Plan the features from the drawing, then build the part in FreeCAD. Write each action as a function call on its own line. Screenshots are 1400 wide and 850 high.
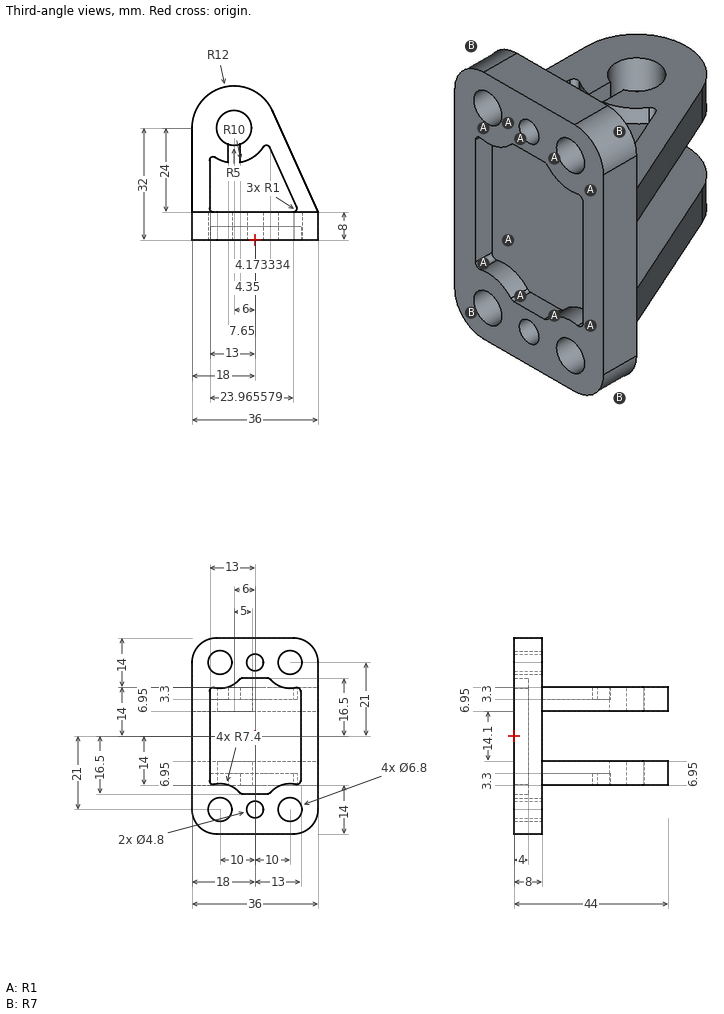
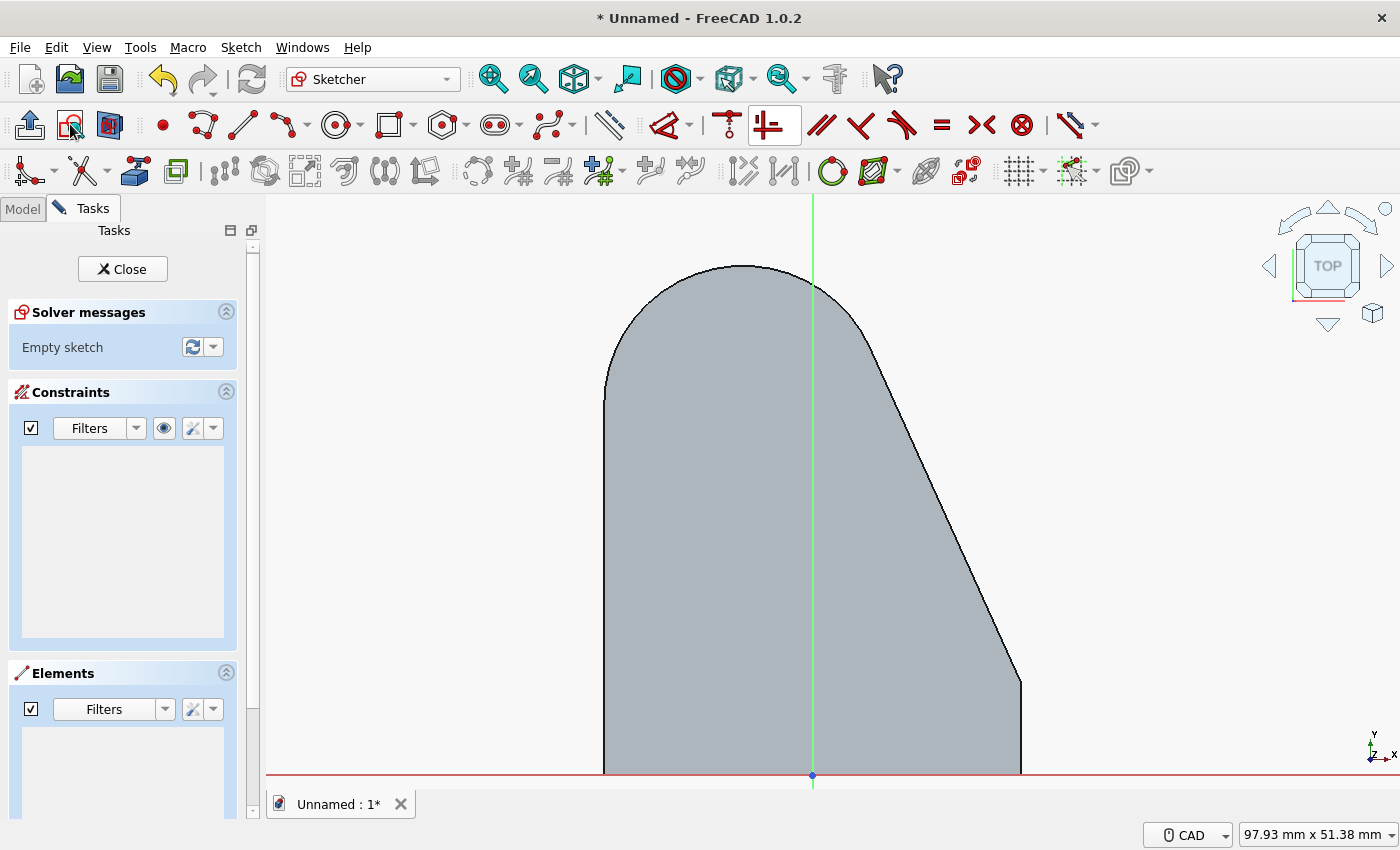
scroll(547, 222, down, 1)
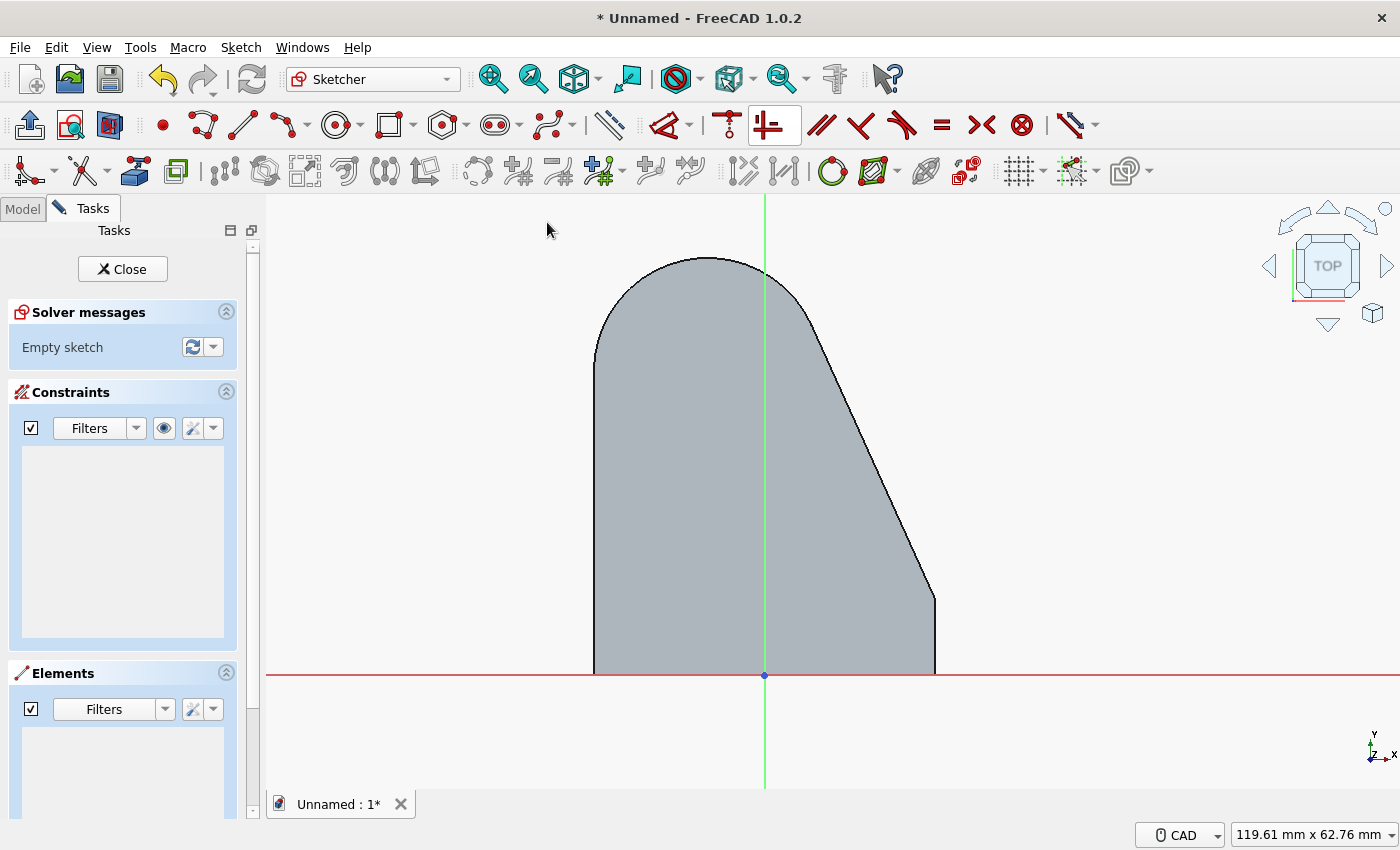
scroll(765, 761, up, 3)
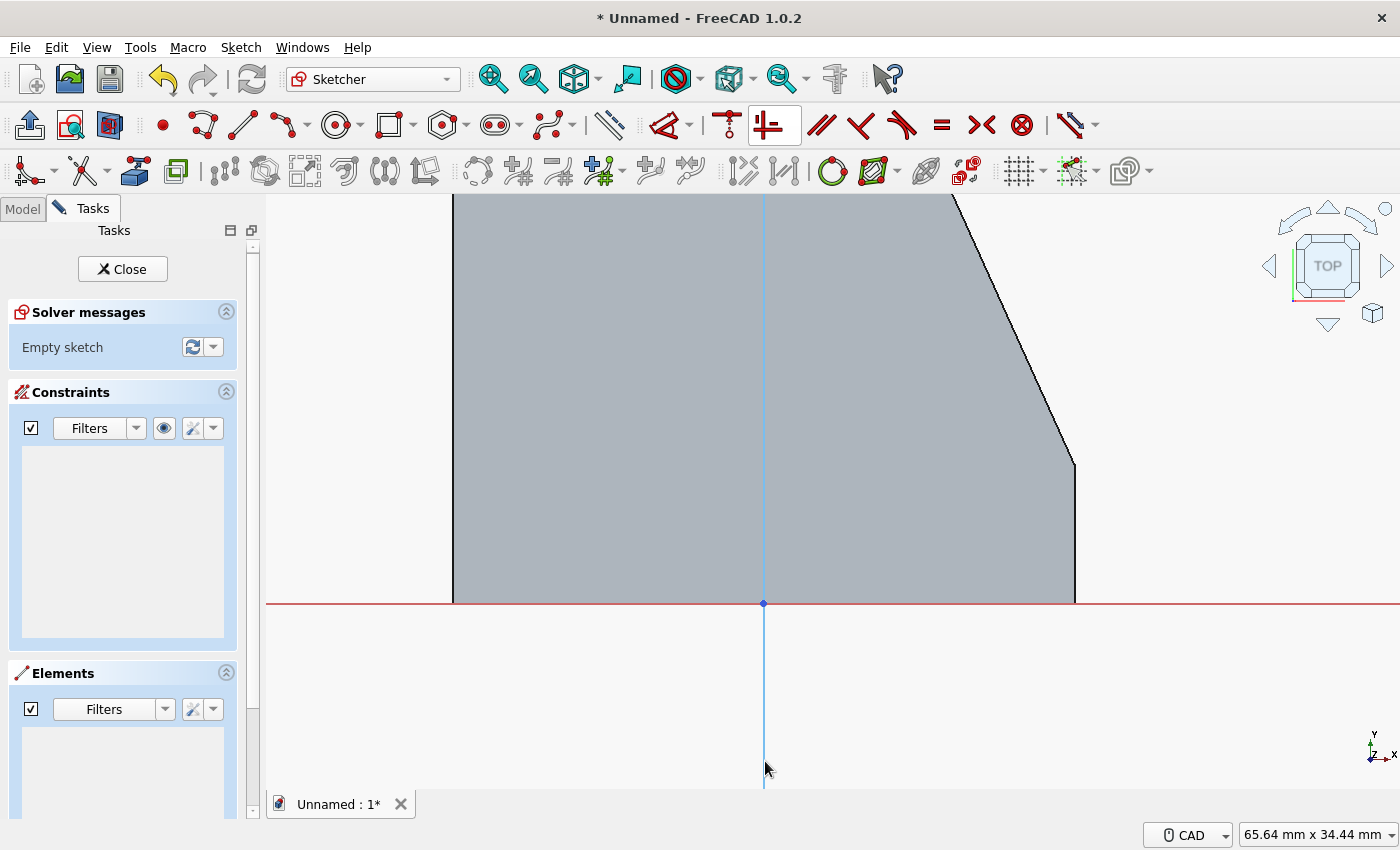
key(g)
key(r)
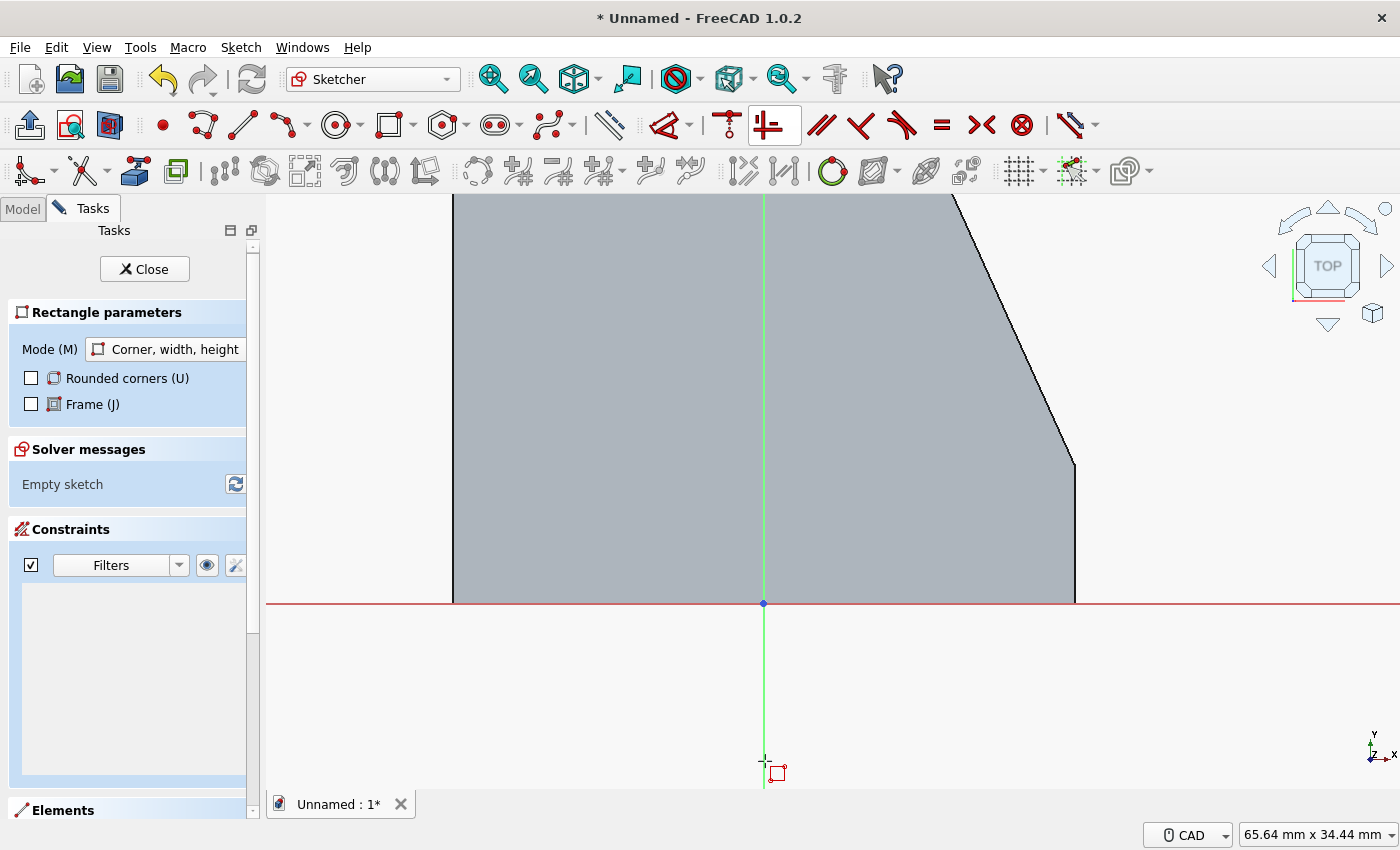
click(453, 465)
click(1075, 604)
key(Escape)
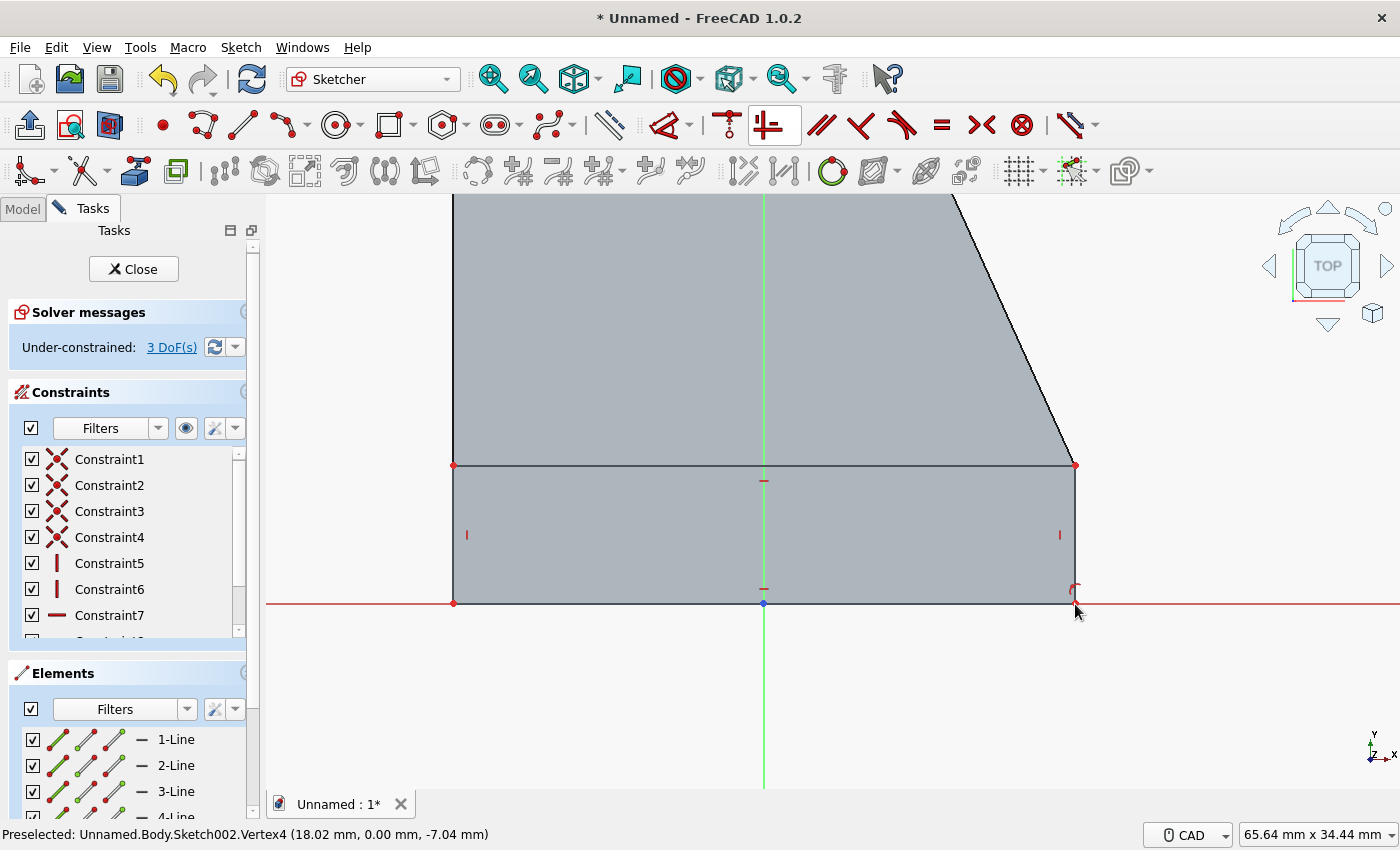
click(453, 507)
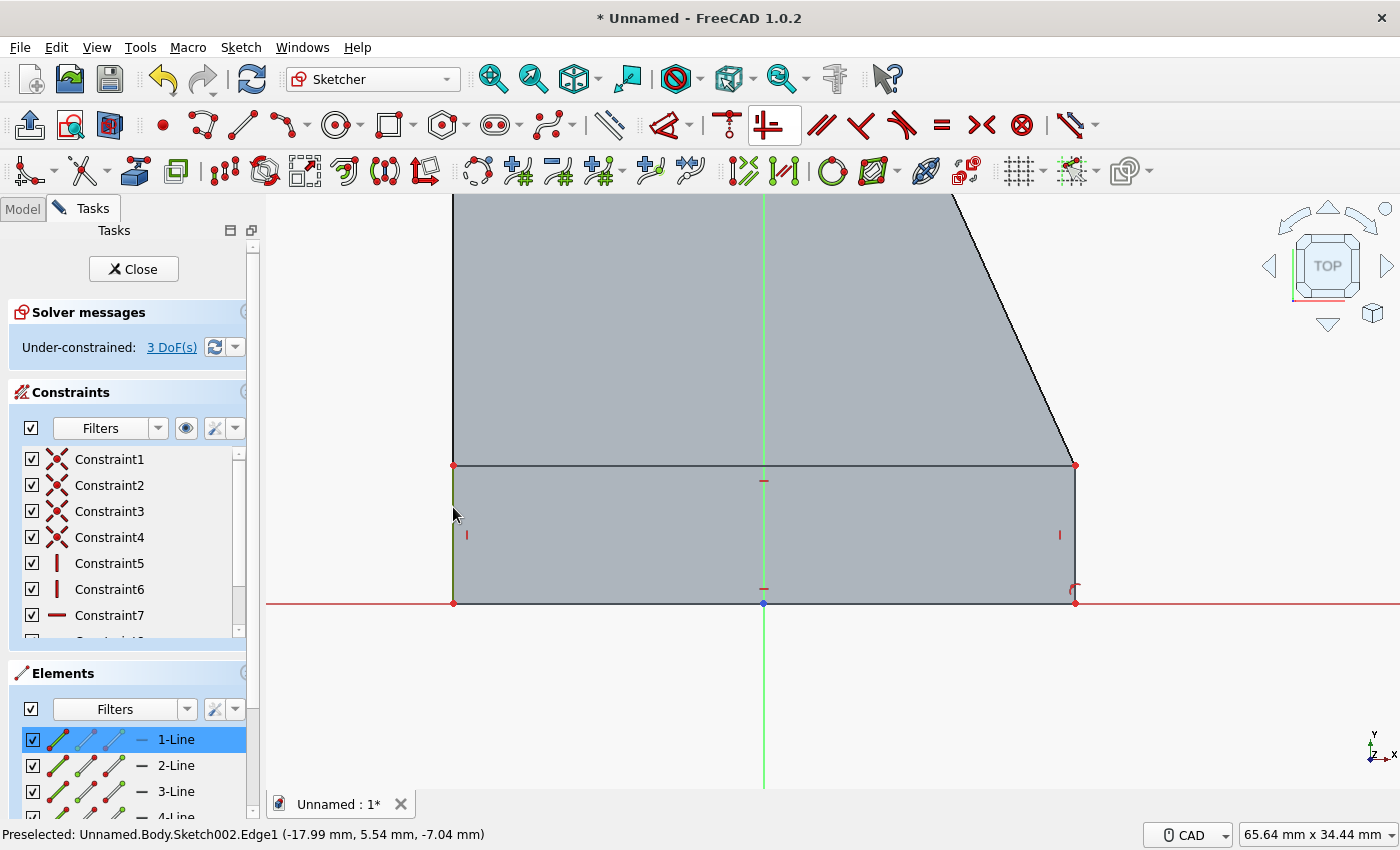
key(i)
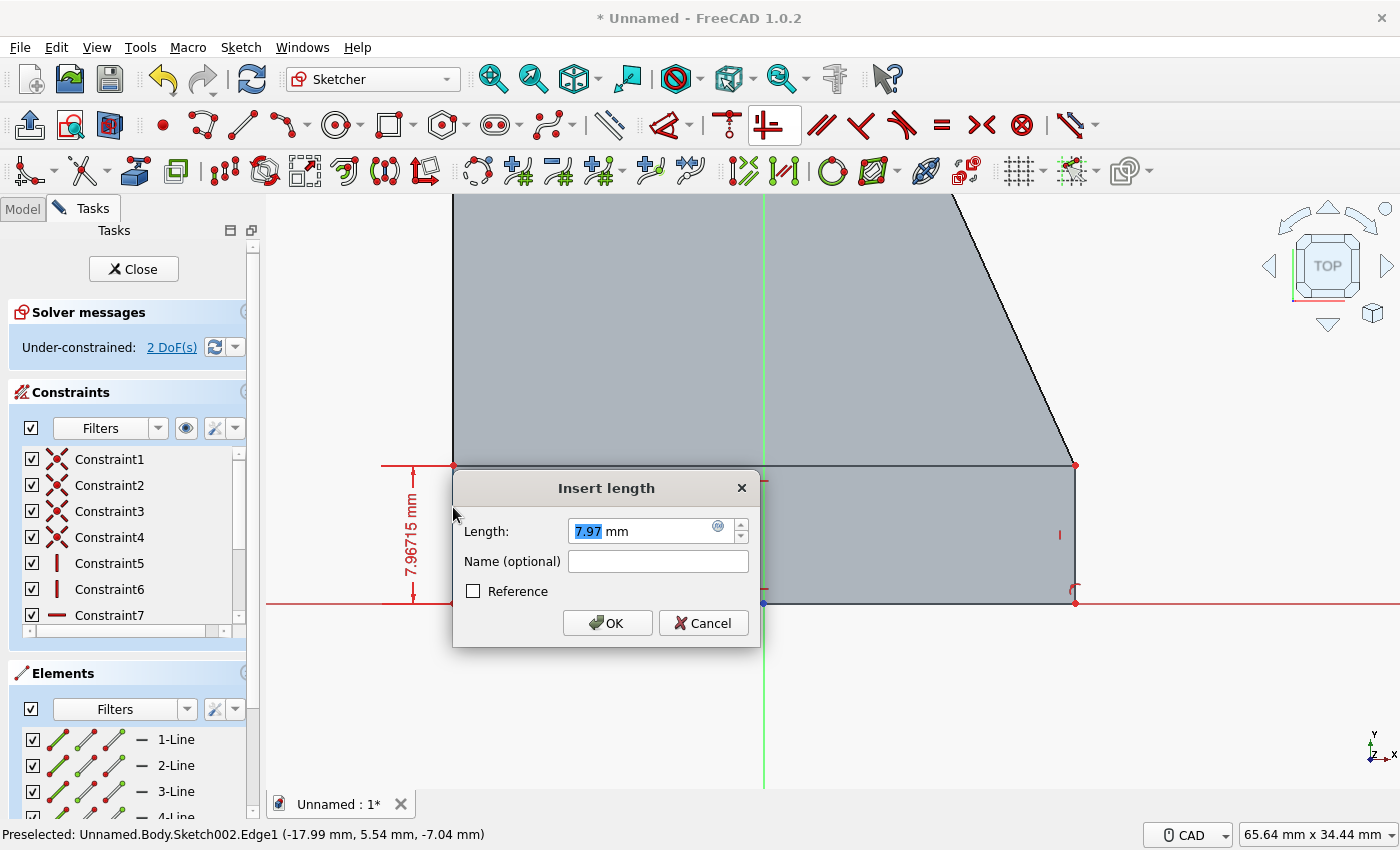
text(8)
key(Return)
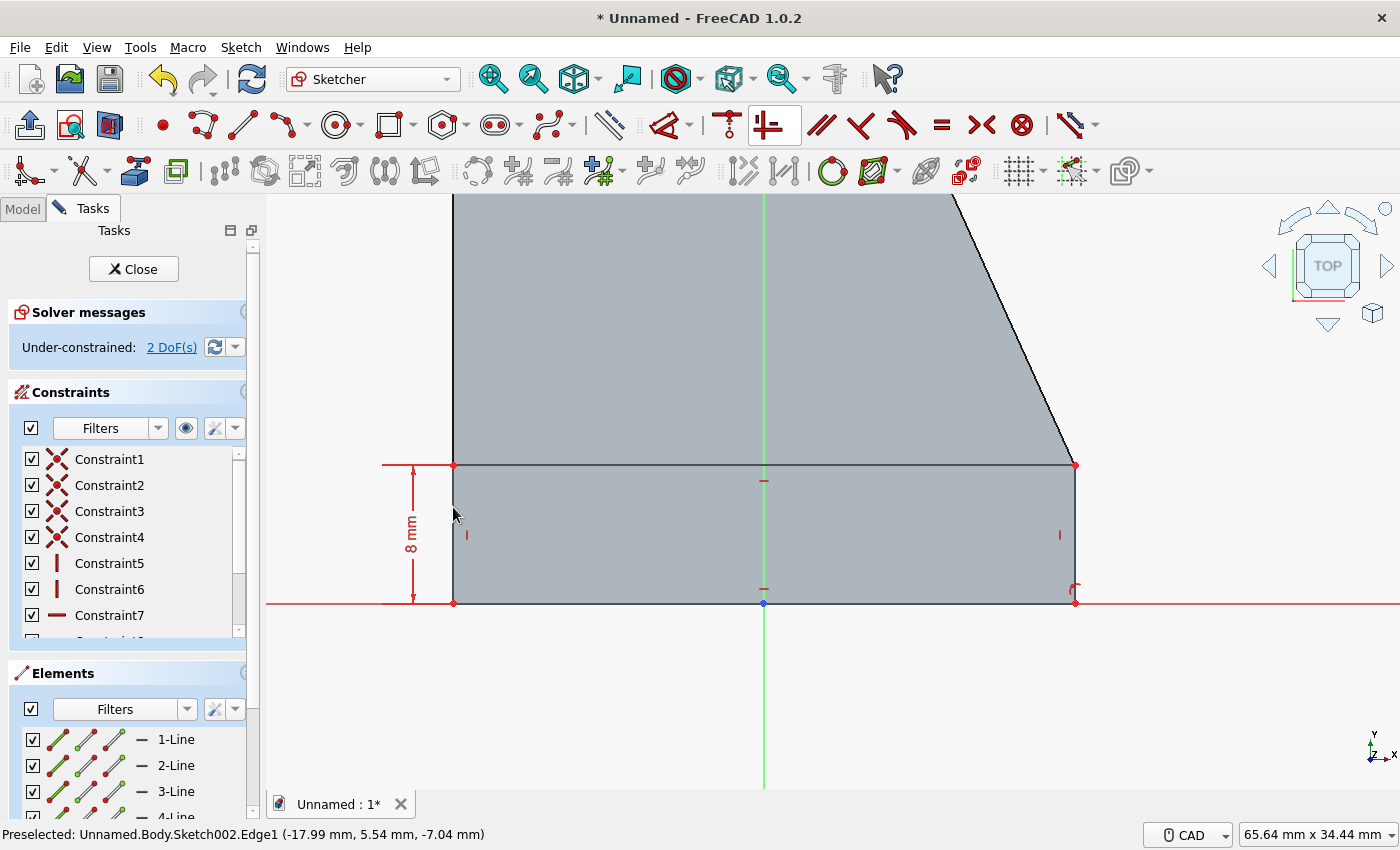
click(640, 604)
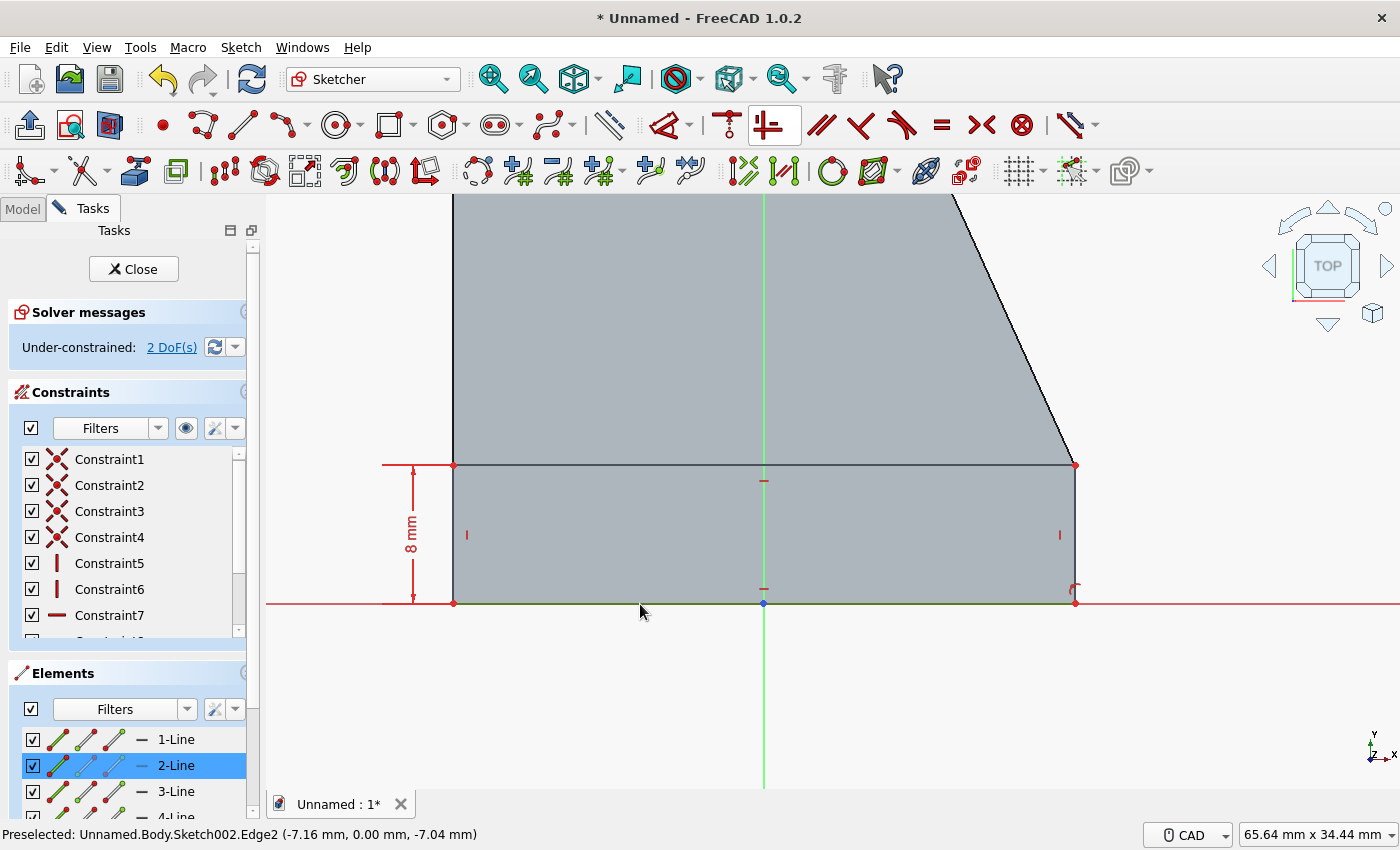
key(l)